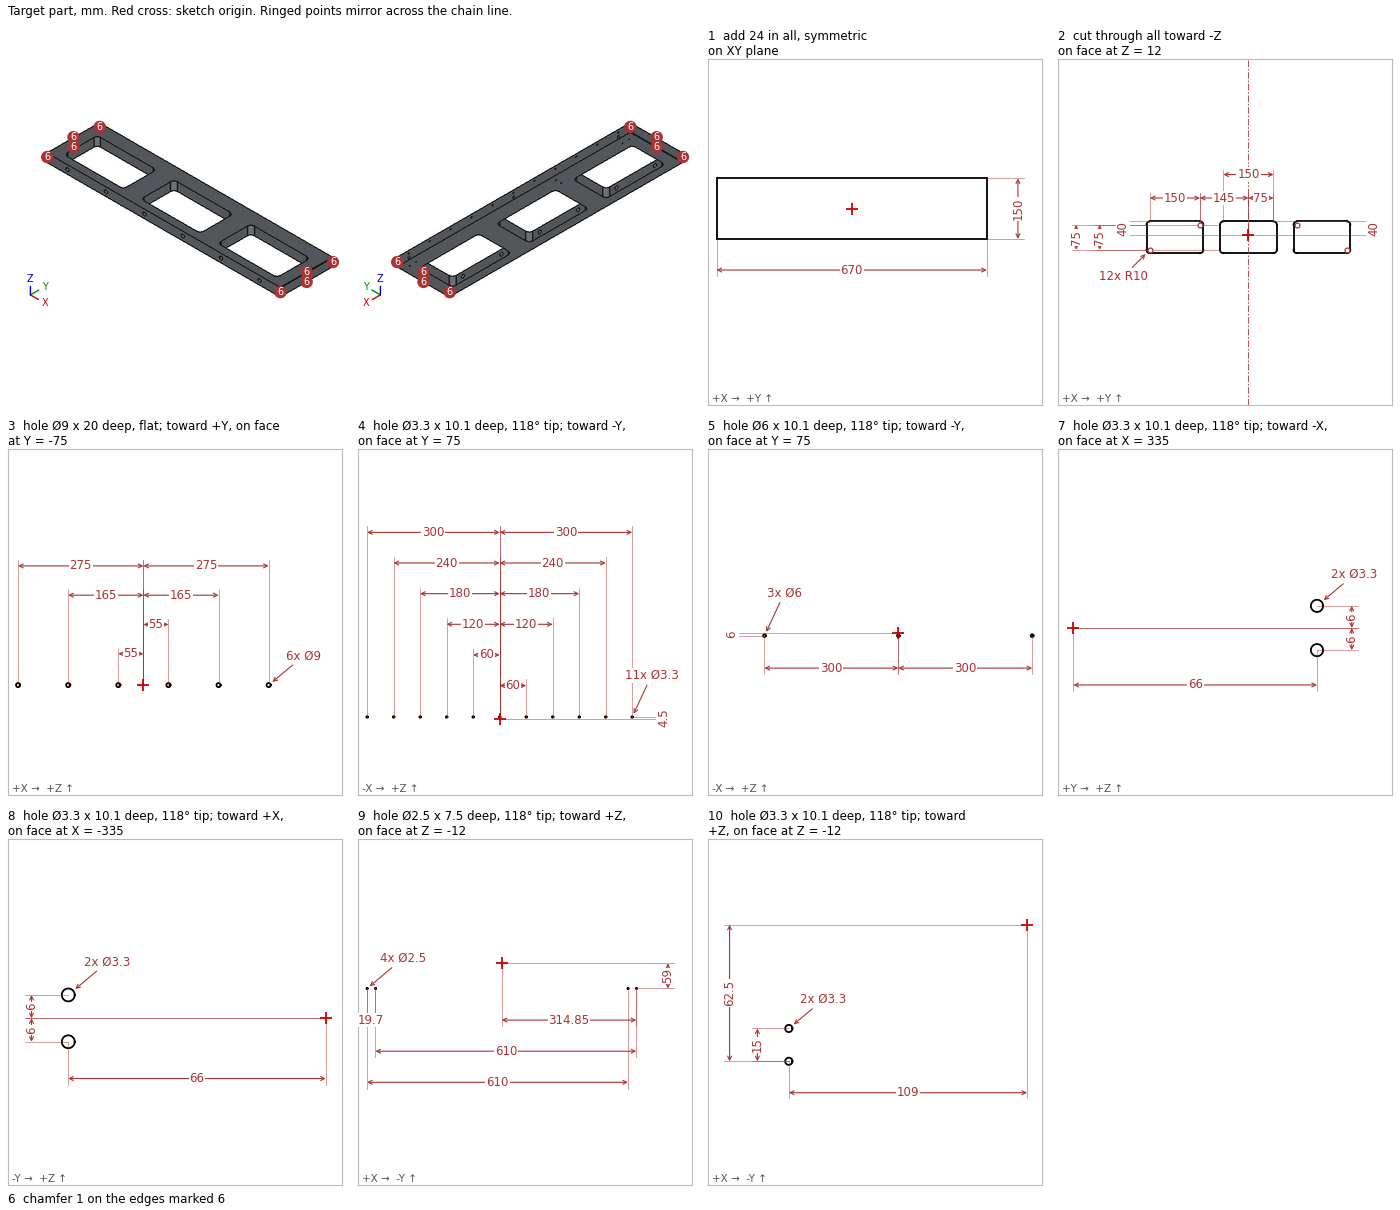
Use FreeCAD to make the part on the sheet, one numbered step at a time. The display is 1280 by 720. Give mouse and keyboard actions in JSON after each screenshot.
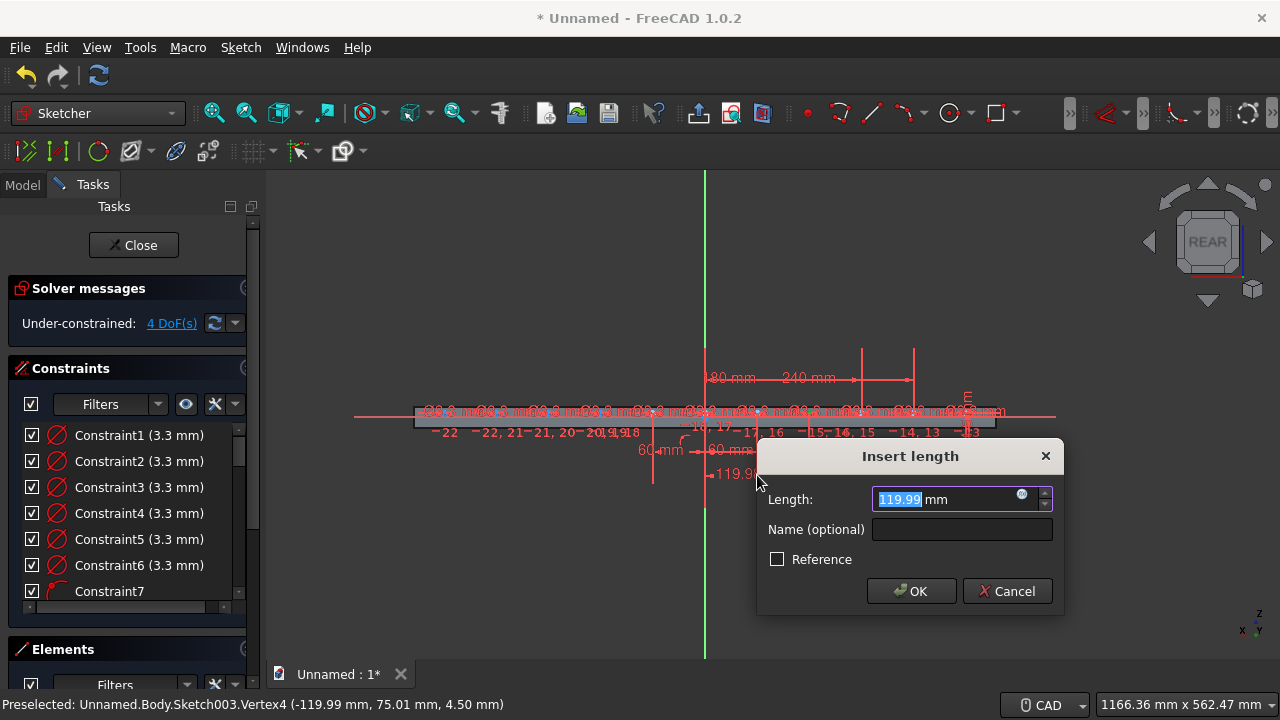
{"action": "type", "text": "120"}
{"action": "key", "text": "Return"}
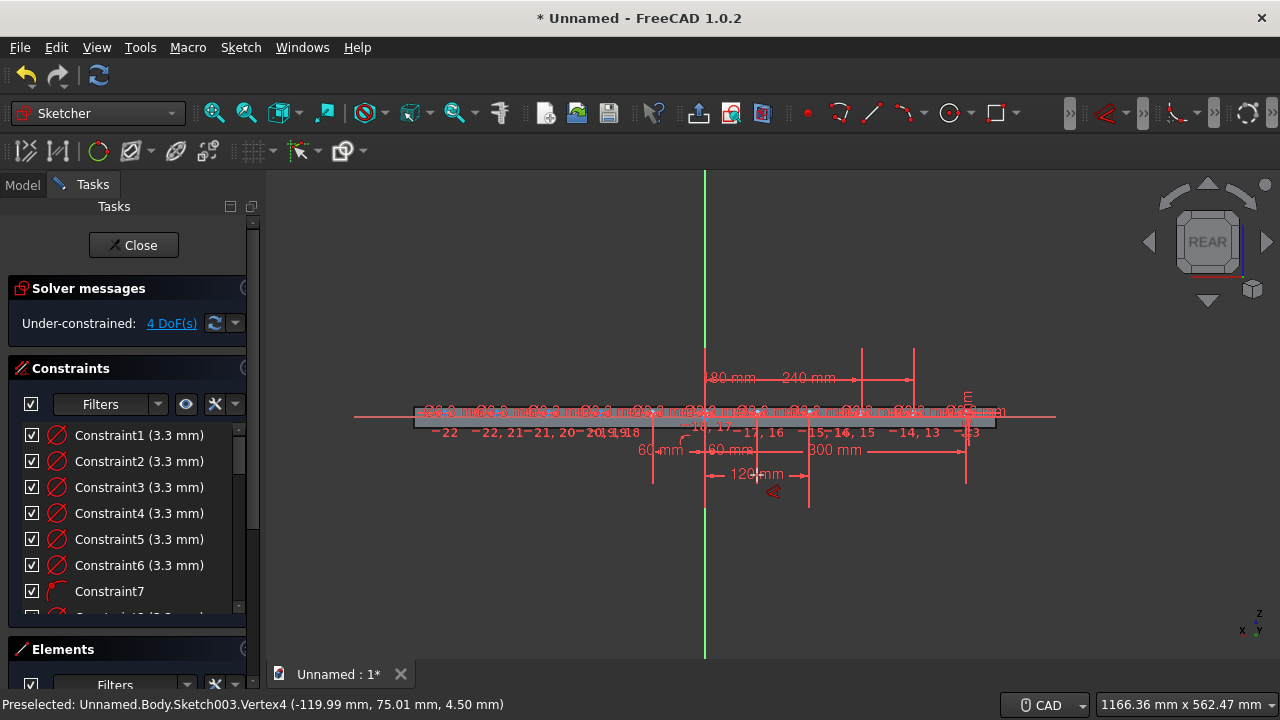
{"action": "left_click", "coordinate": [601, 413]}
{"action": "left_click", "coordinate": [653, 379]}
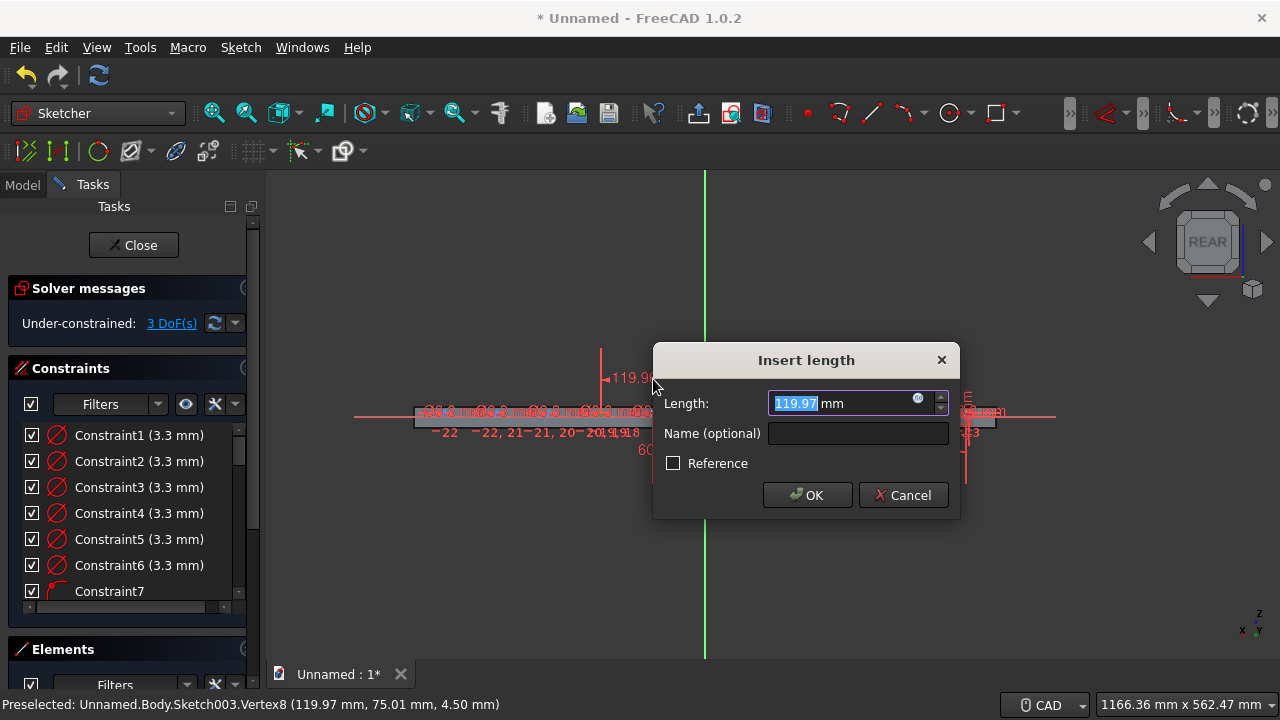
{"action": "type", "text": "120"}
{"action": "key", "text": "Return"}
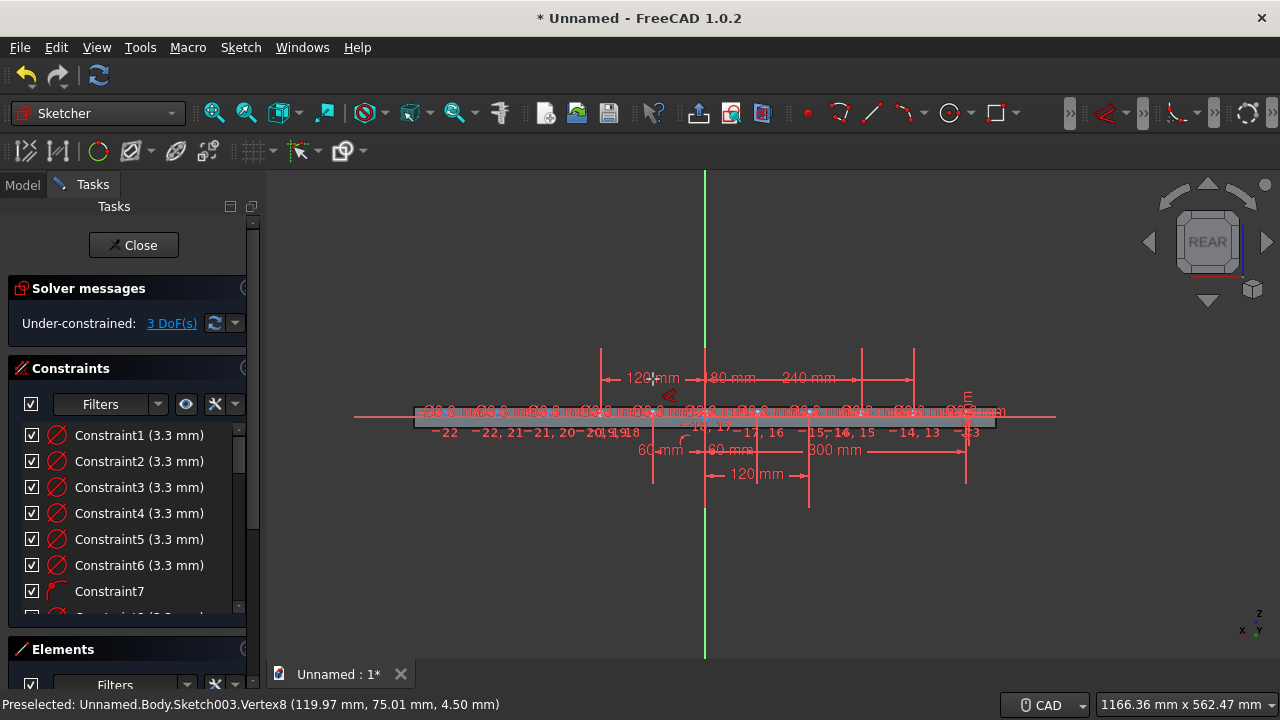
{"action": "left_click", "coordinate": [549, 413]}
{"action": "left_click", "coordinate": [572, 451]}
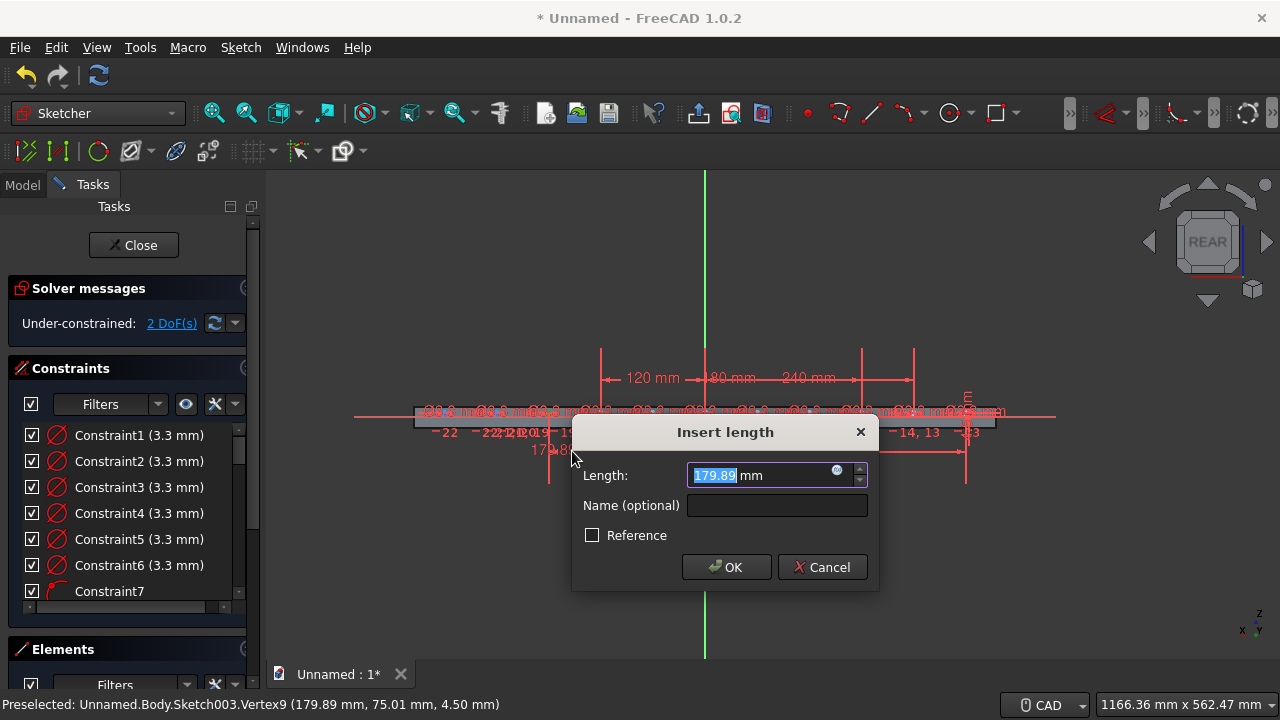
{"action": "type", "text": "180"}
{"action": "key", "text": "Return"}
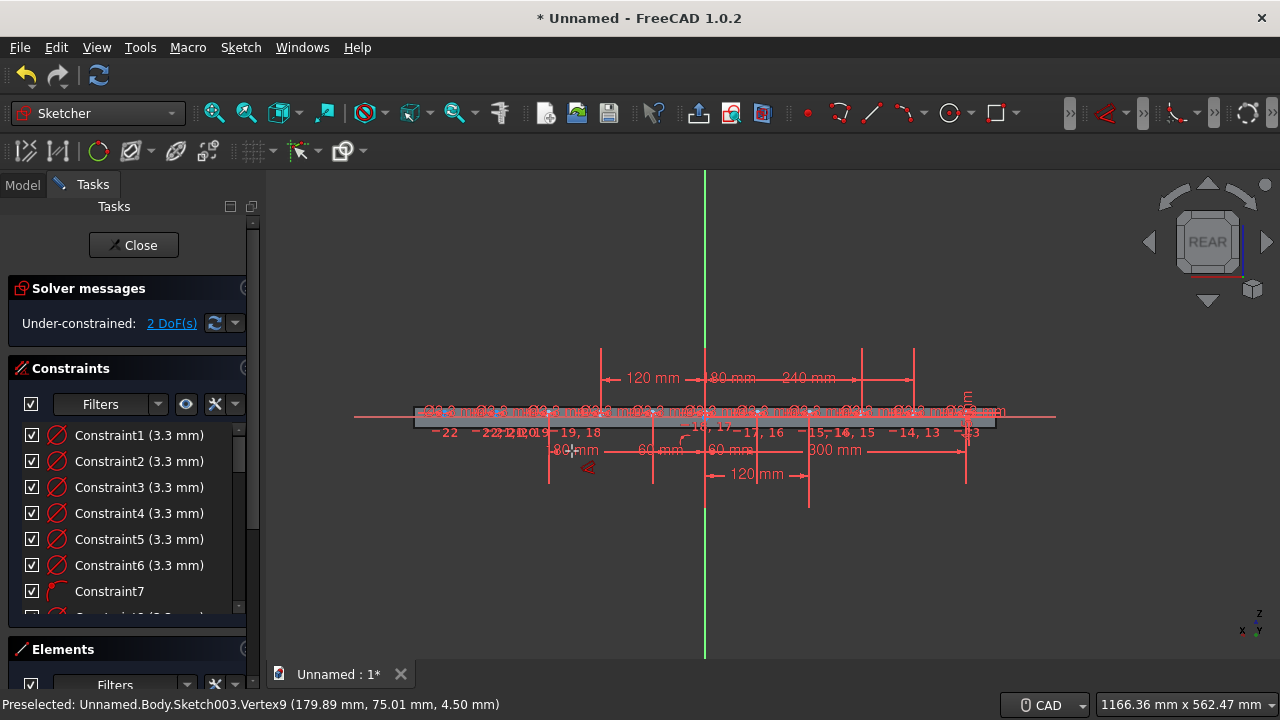
{"action": "left_click", "coordinate": [496, 413]}
{"action": "left_click", "coordinate": [553, 379]}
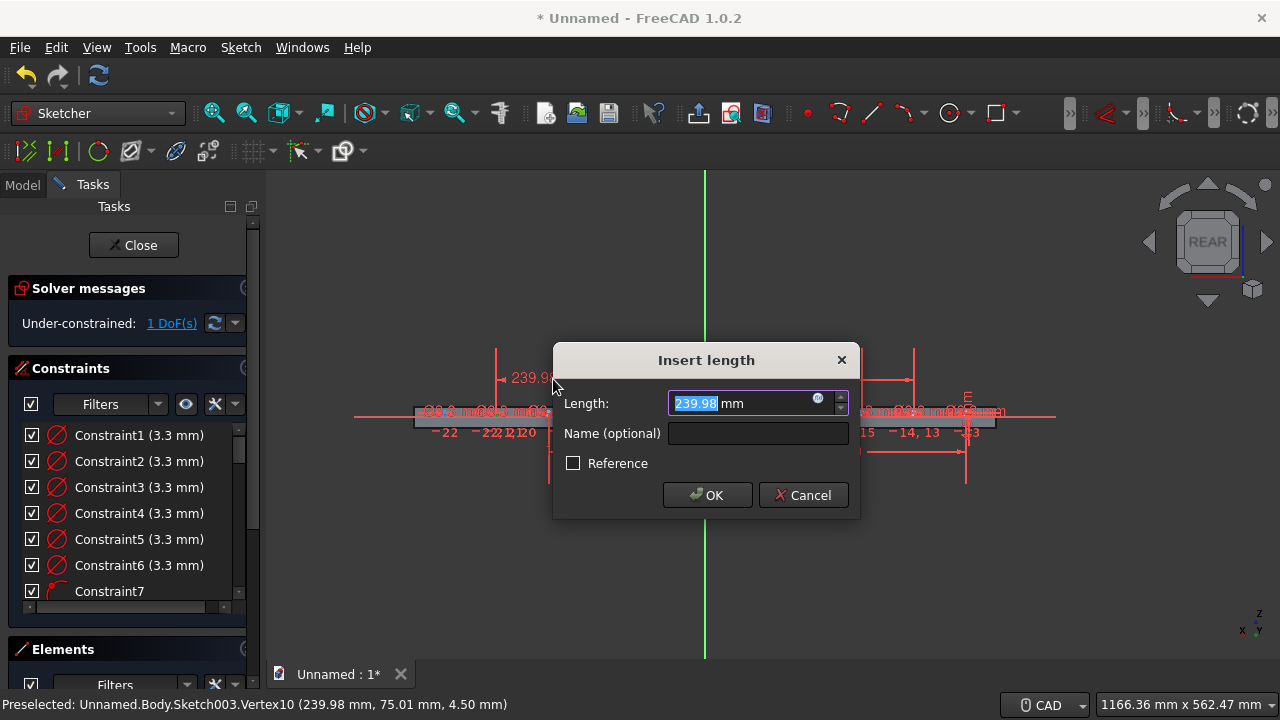
{"action": "type", "text": "240"}
{"action": "key", "text": "Return"}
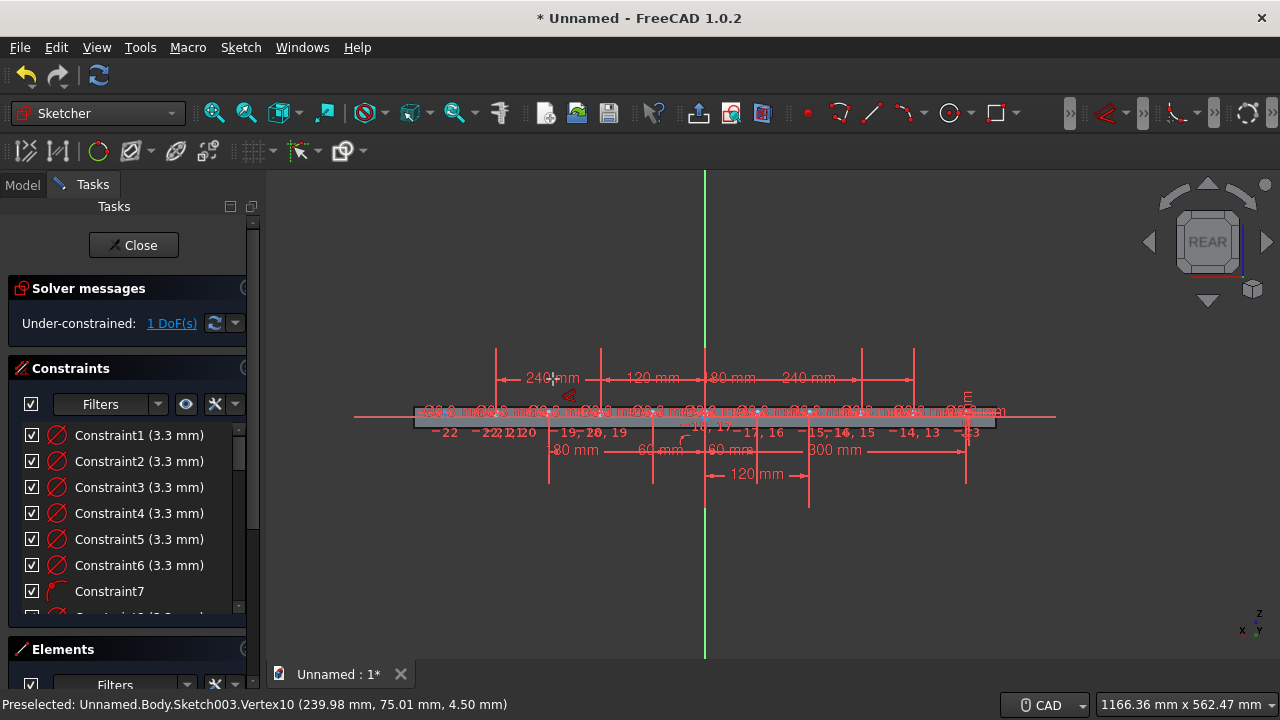
{"action": "left_click", "coordinate": [444, 413]}
{"action": "left_click", "coordinate": [483, 451]}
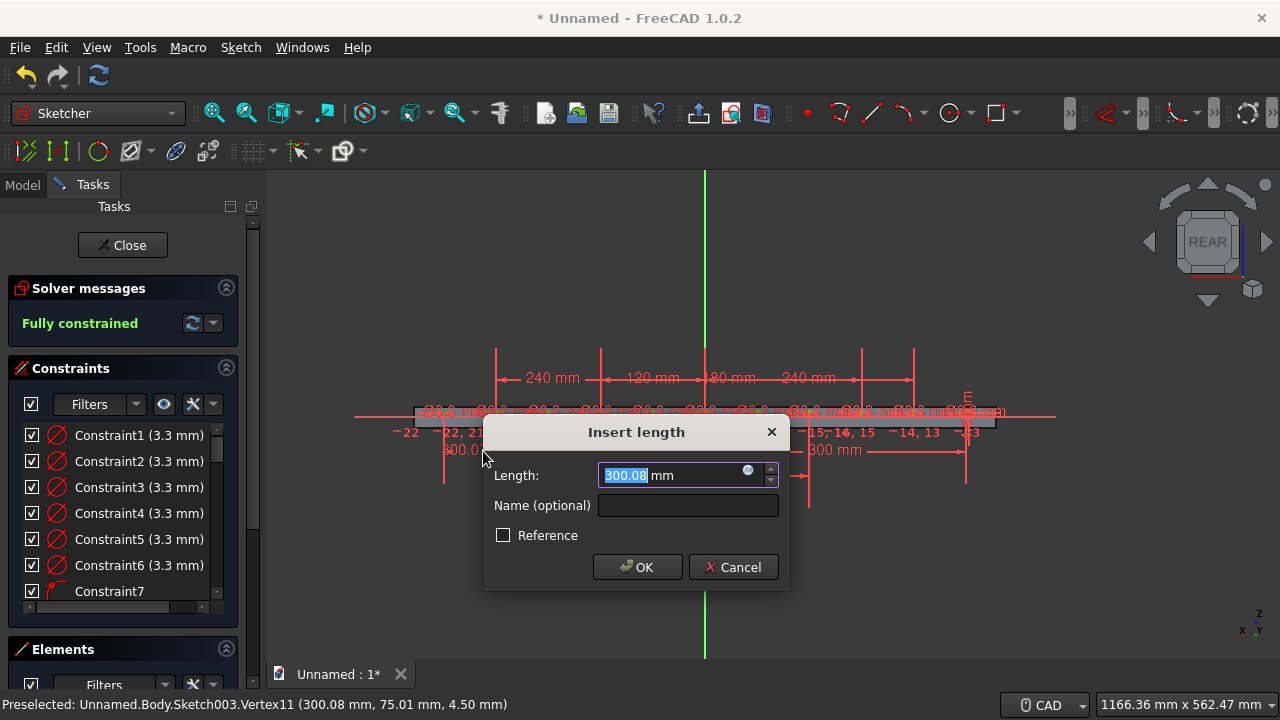
{"action": "type", "text": "300"}
{"action": "key", "text": "Return"}
{"action": "key", "text": "Escape"}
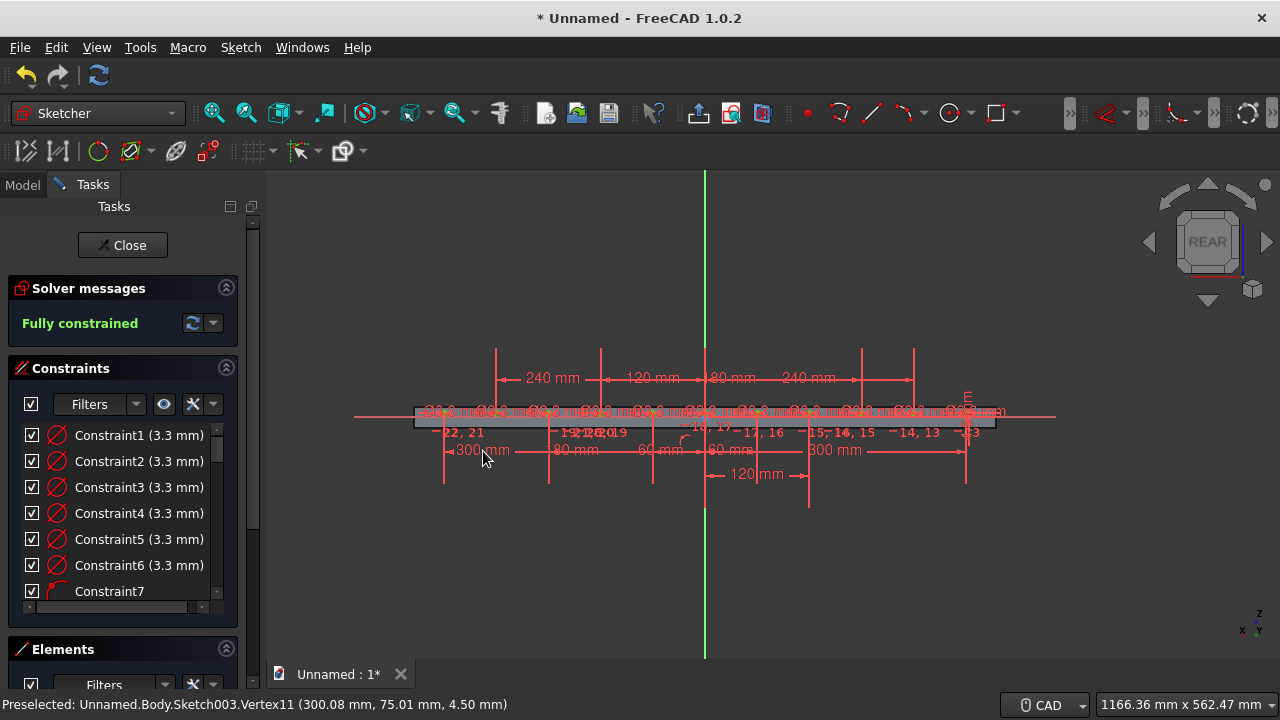
{"action": "left_click", "coordinate": [123, 245]}